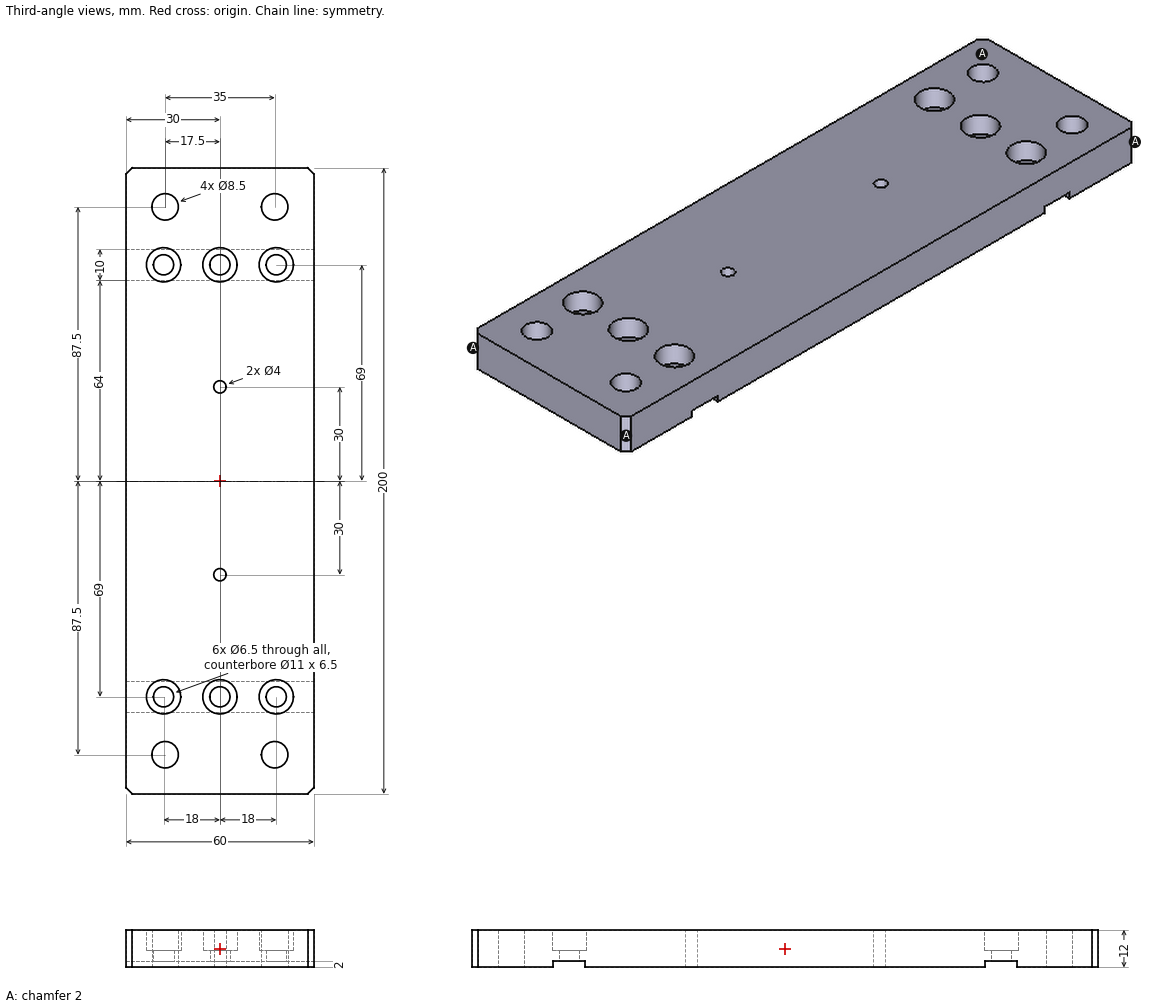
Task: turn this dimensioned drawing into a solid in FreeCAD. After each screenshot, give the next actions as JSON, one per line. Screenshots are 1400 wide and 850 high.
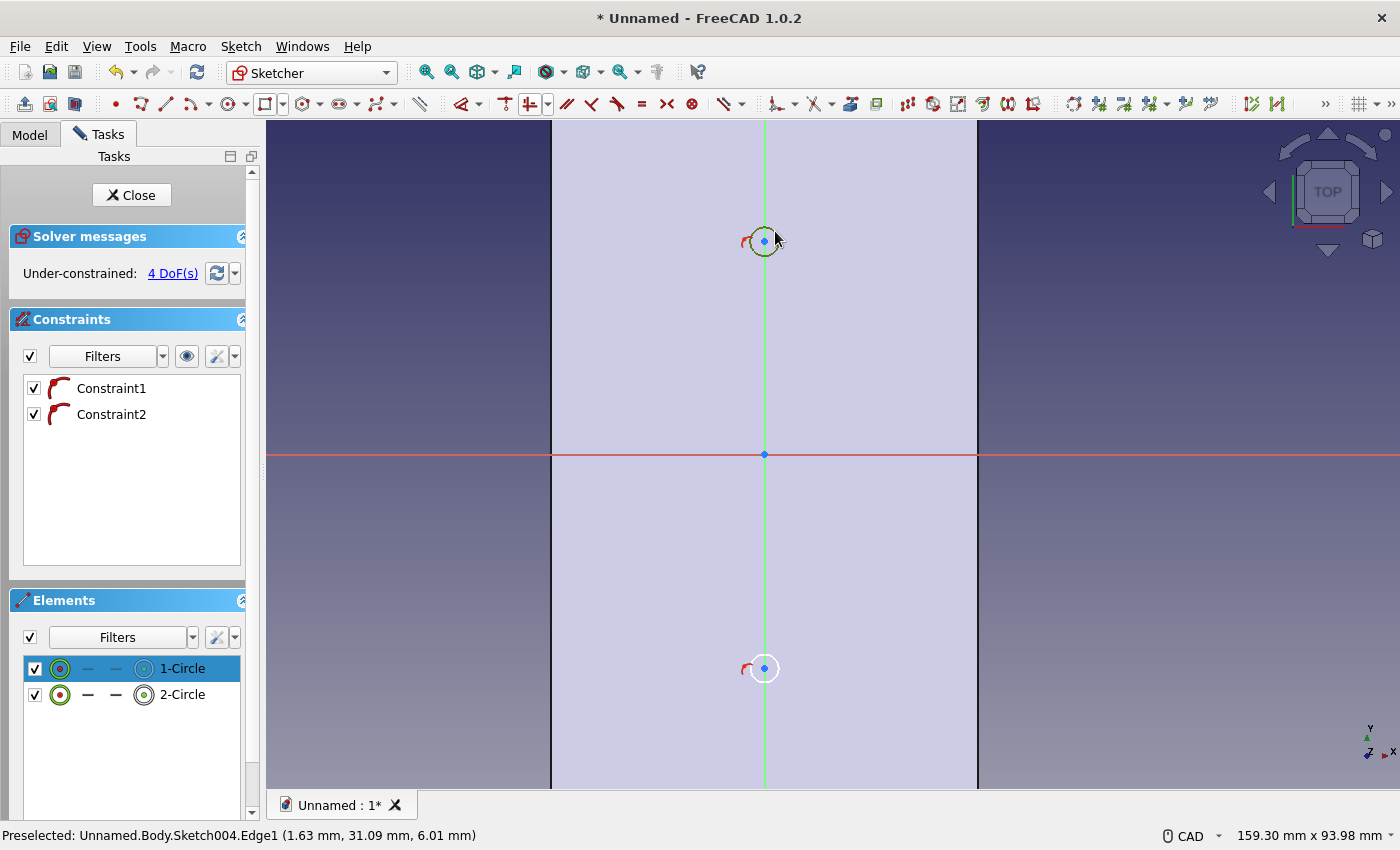
{"action": "scroll", "coordinate": [774, 659], "scroll_direction": "up", "scroll_amount": 2}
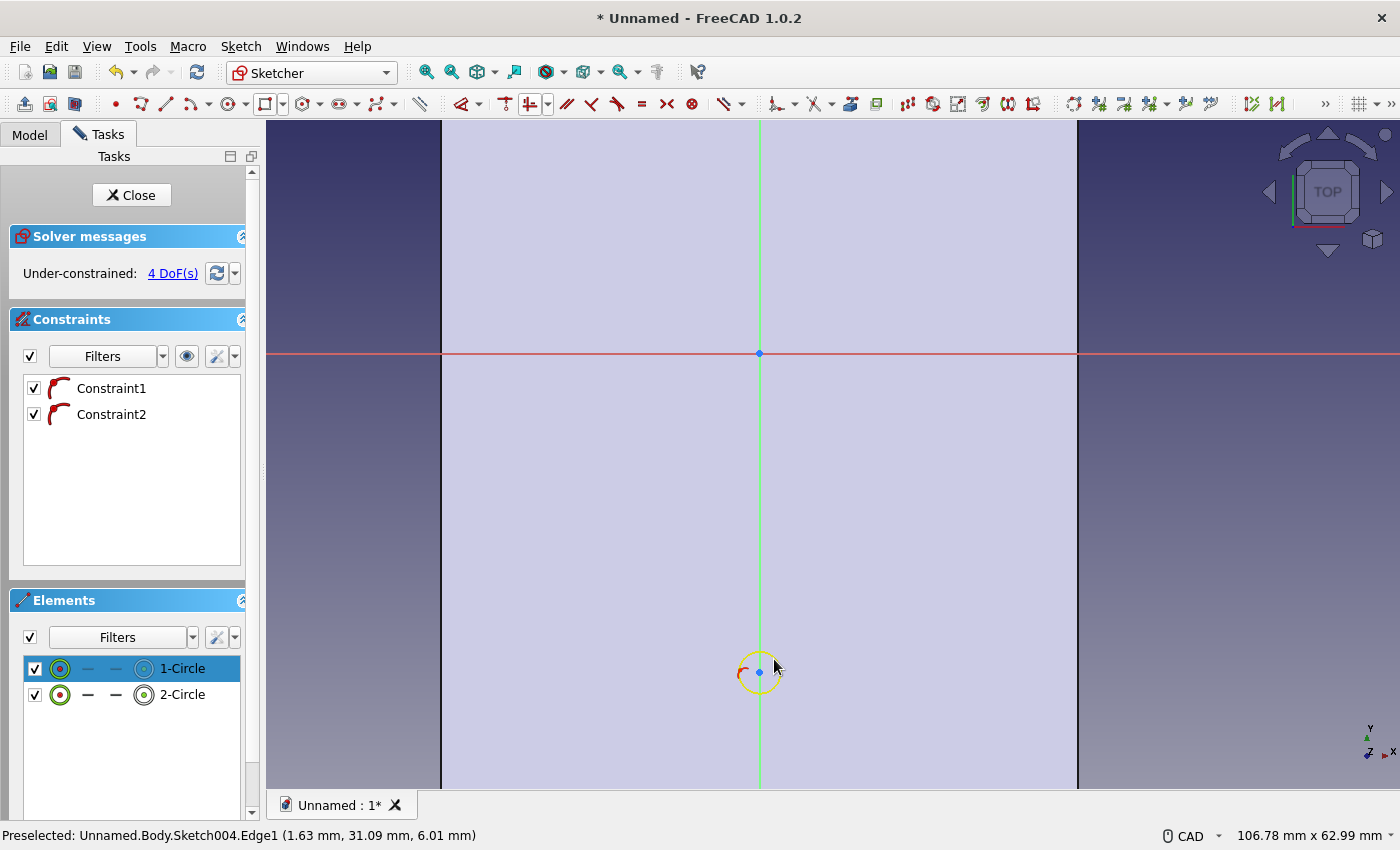
{"action": "left_click", "coordinate": [774, 658]}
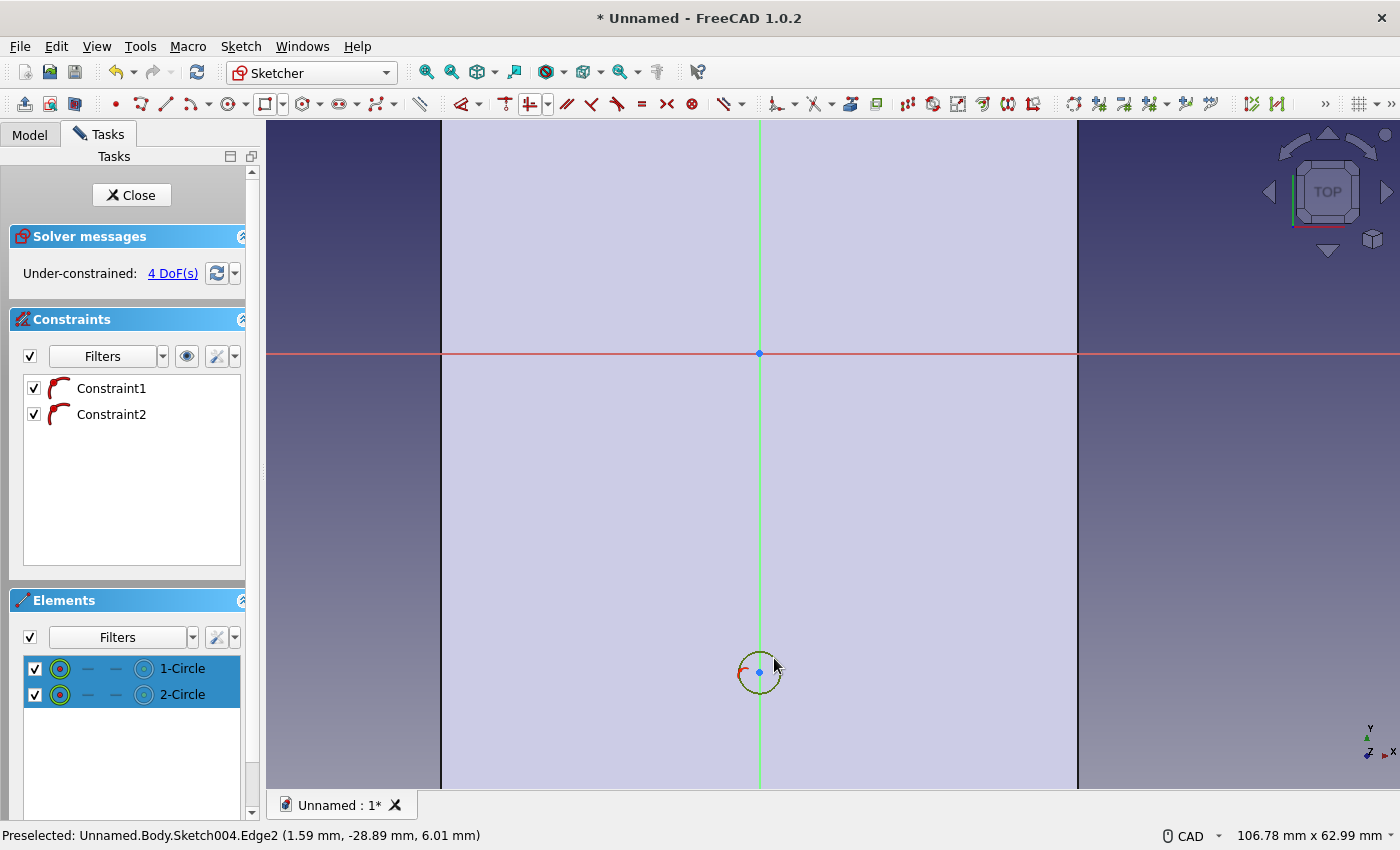
{"action": "left_click", "coordinate": [642, 104]}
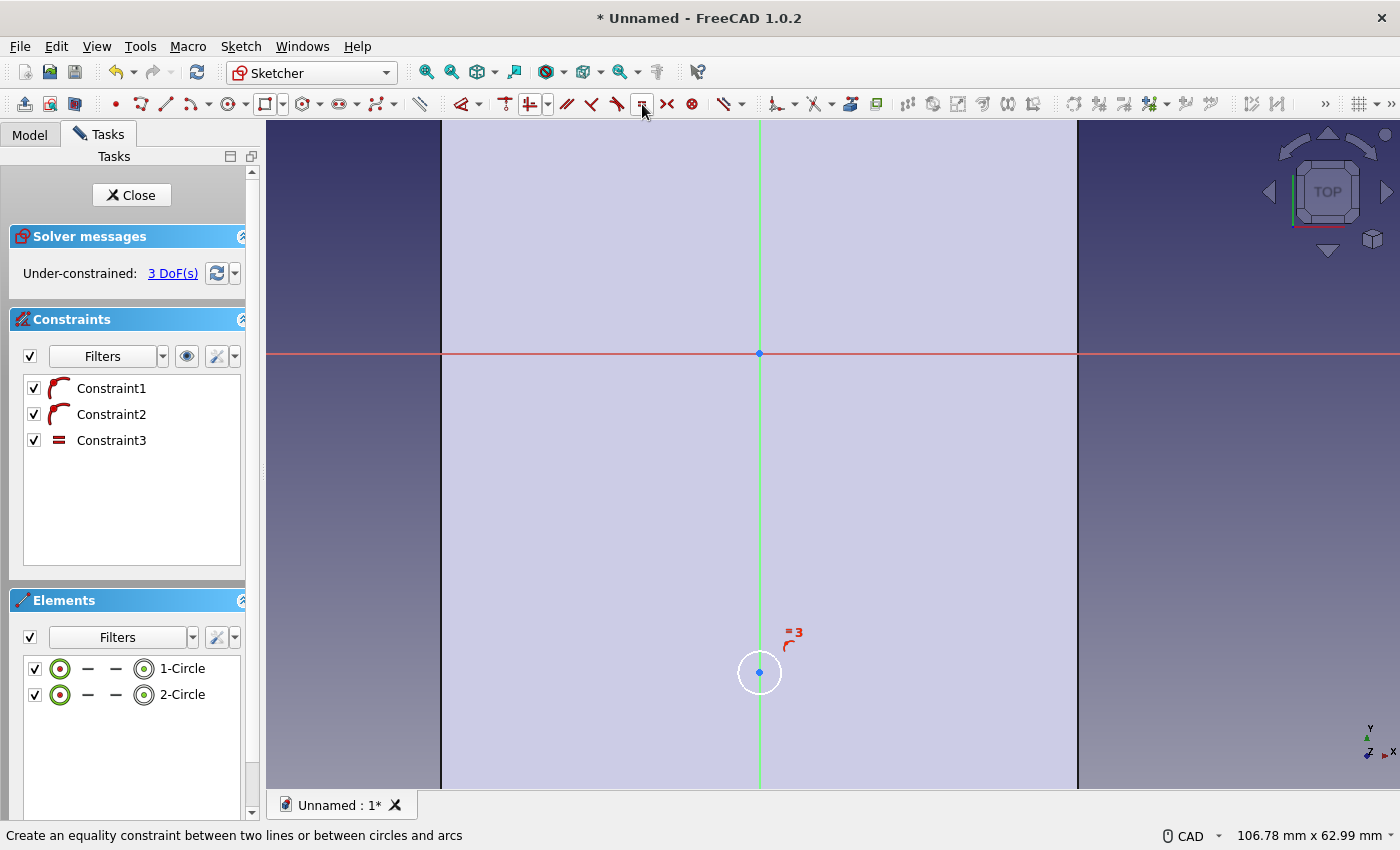
{"action": "left_click", "coordinate": [460, 104]}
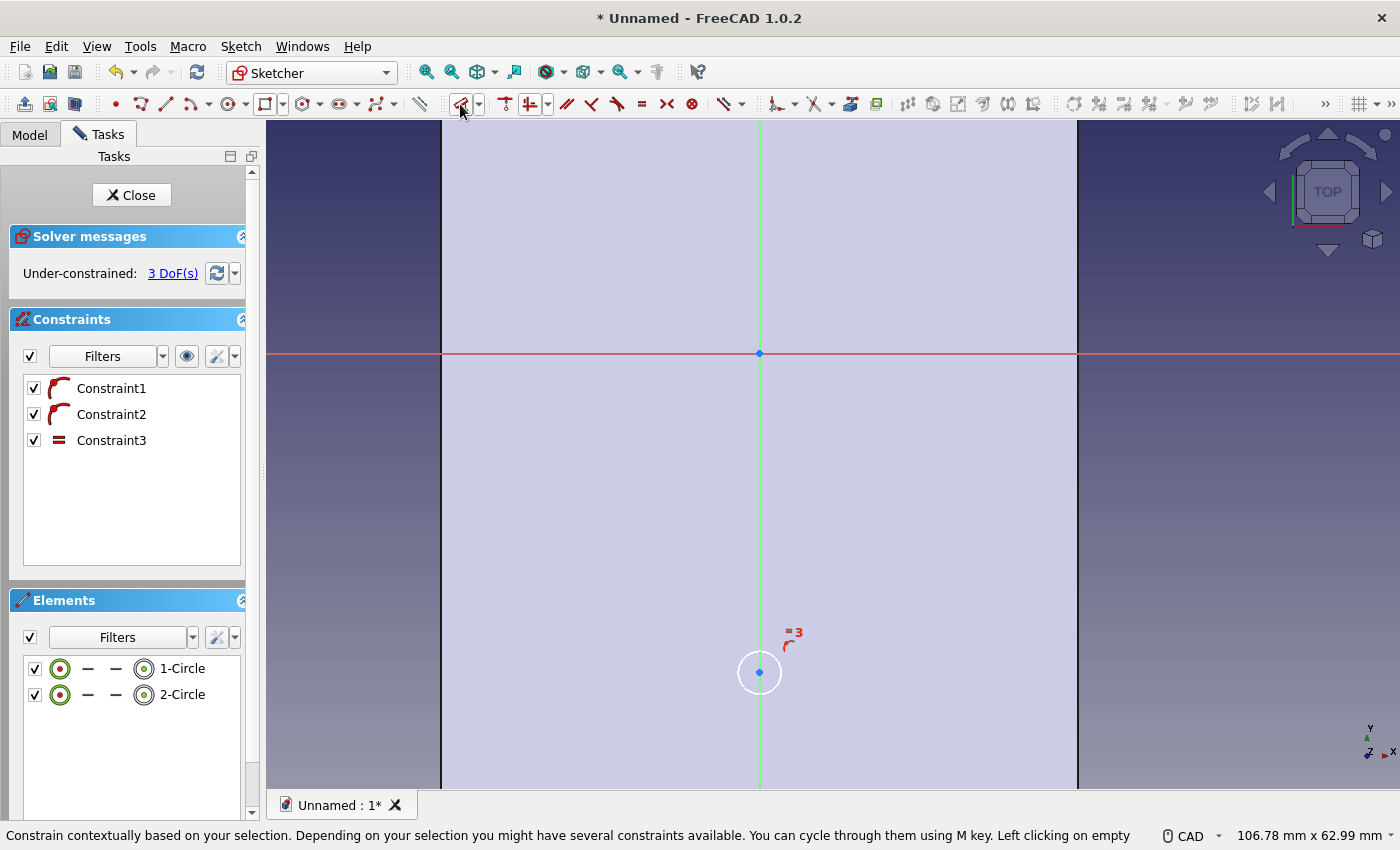
{"action": "scroll", "coordinate": [774, 659], "scroll_direction": "down", "scroll_amount": 2}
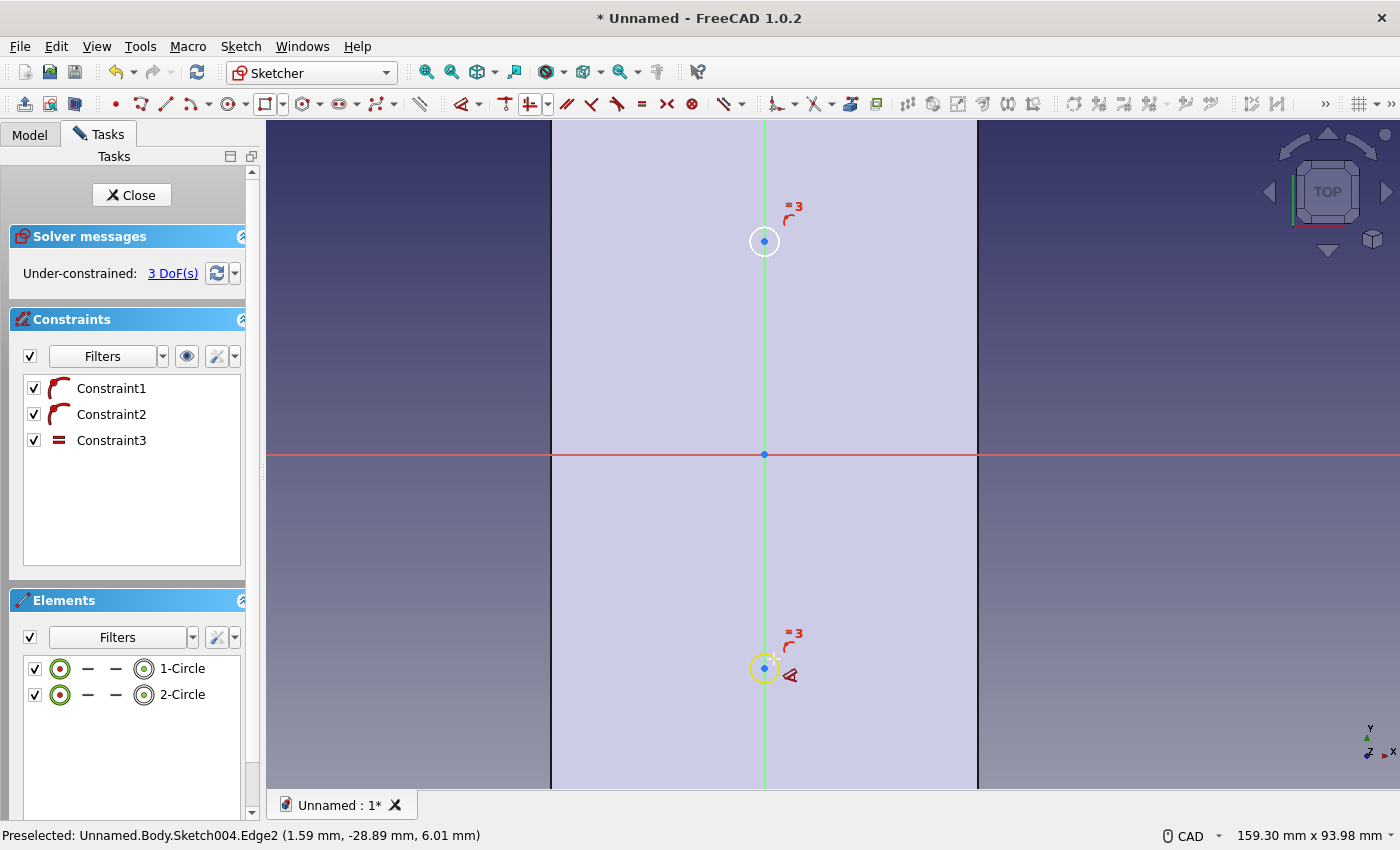
{"action": "scroll", "coordinate": [775, 232], "scroll_direction": "up", "scroll_amount": 2}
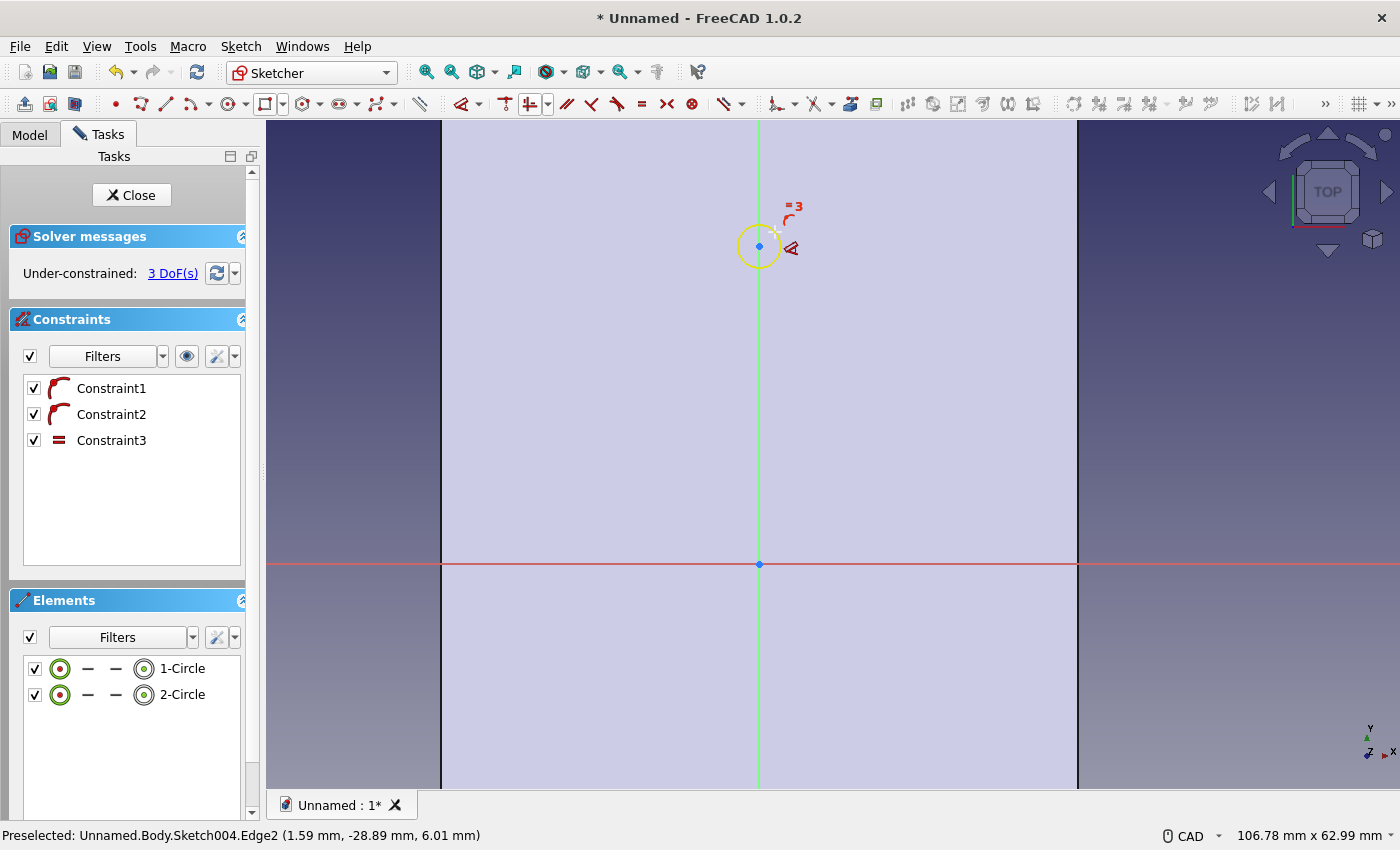
{"action": "left_click", "coordinate": [774, 231]}
{"action": "left_click", "coordinate": [796, 208]}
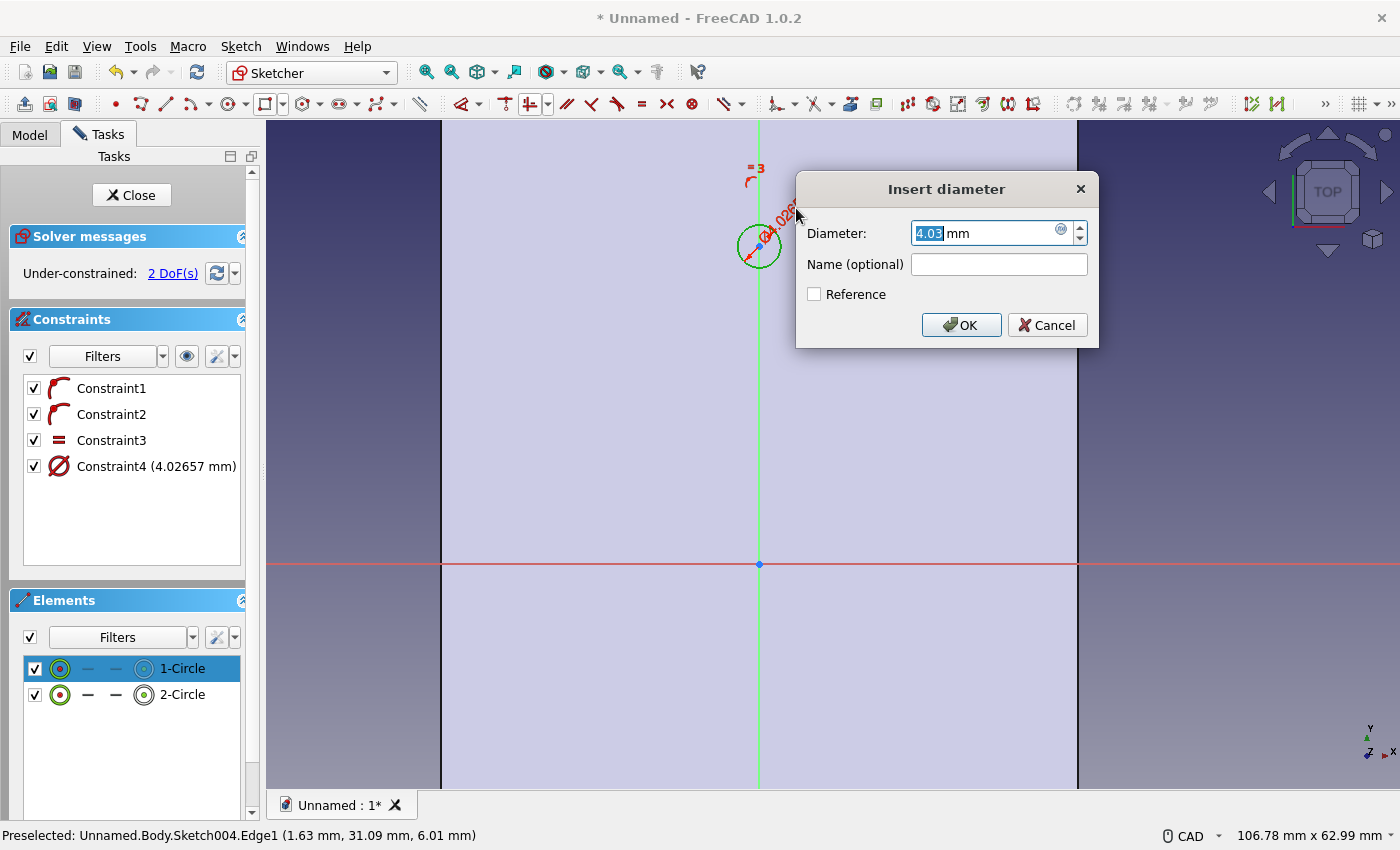
{"action": "type", "text": "4"}
{"action": "key", "text": "Return"}